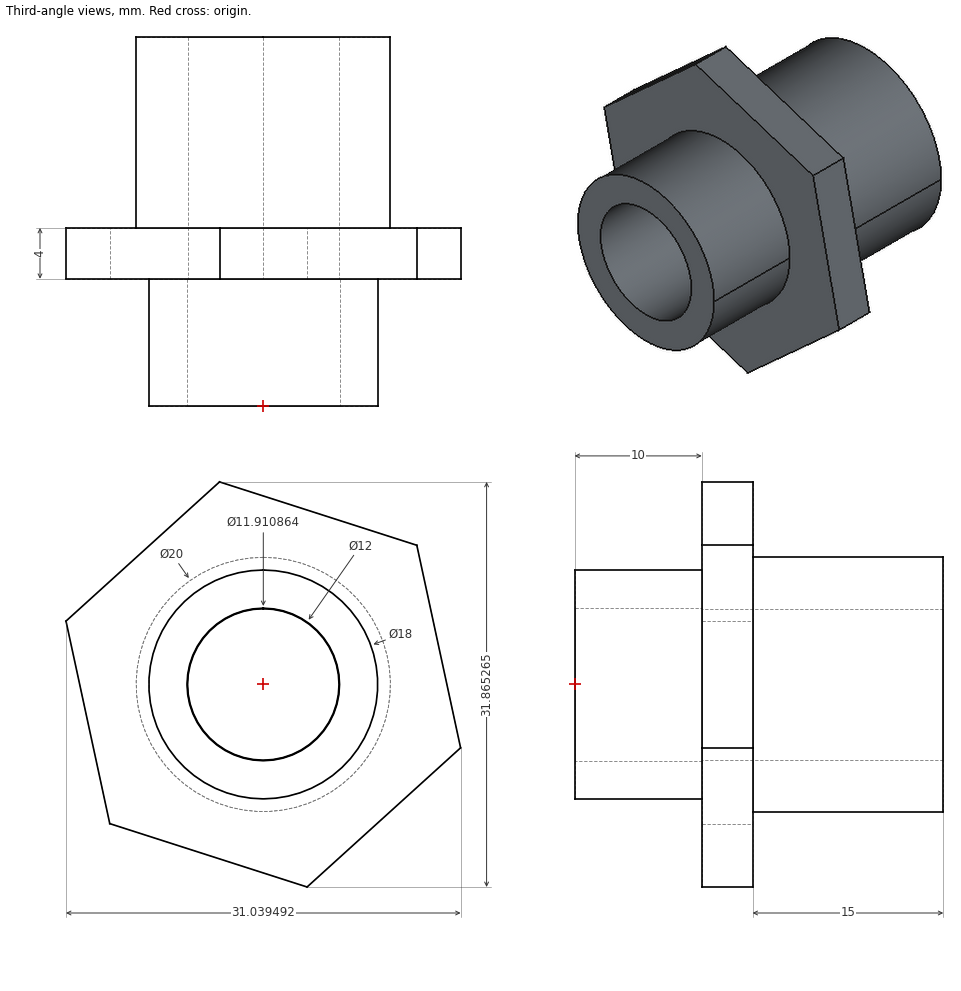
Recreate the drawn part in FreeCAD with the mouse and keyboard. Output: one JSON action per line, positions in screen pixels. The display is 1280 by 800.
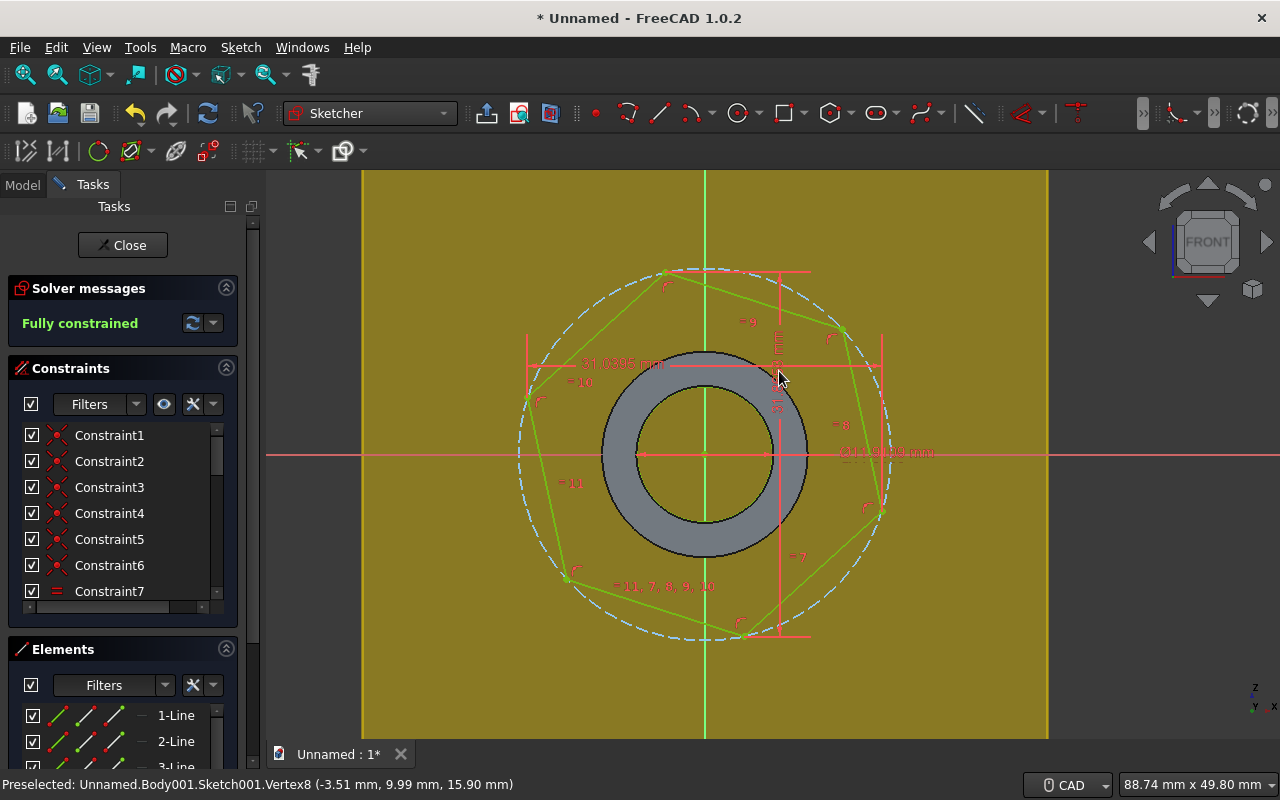
{"action": "left_click", "coordinate": [123, 245]}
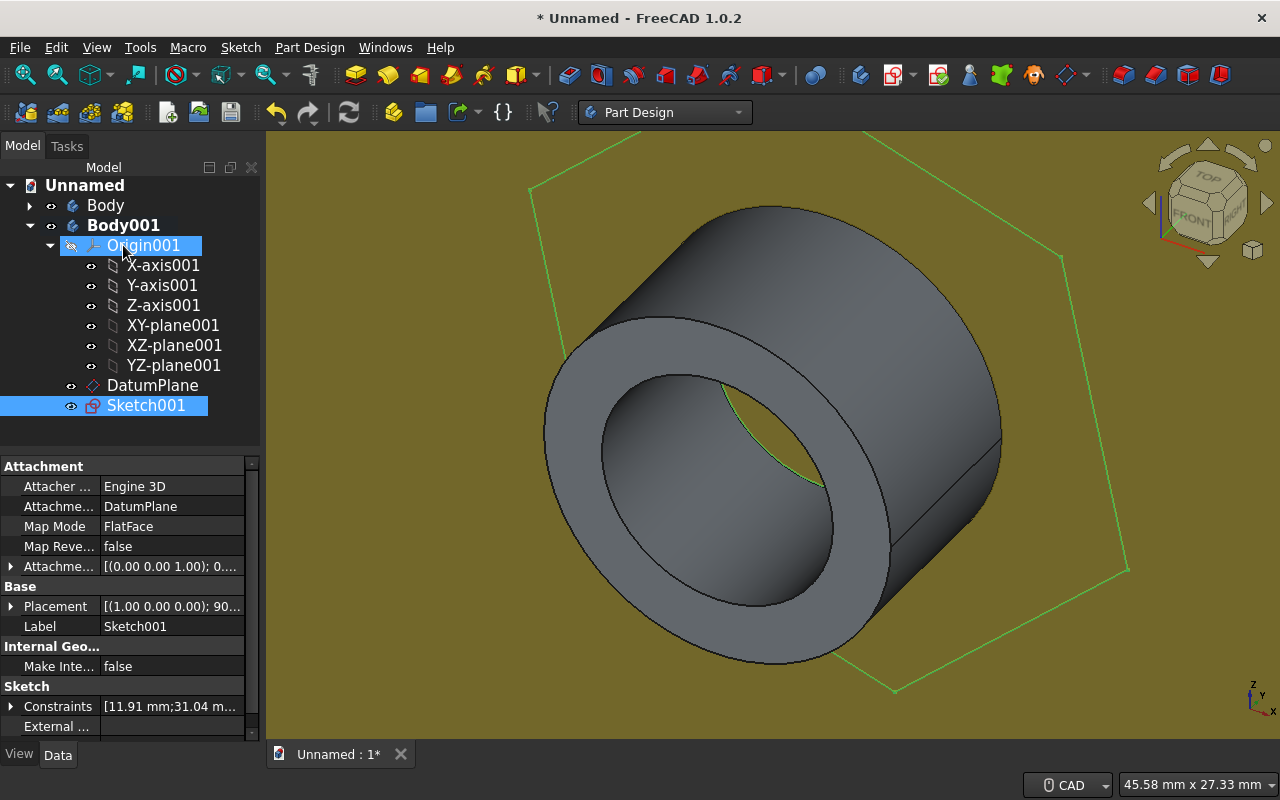
{"action": "left_click", "coordinate": [356, 76]}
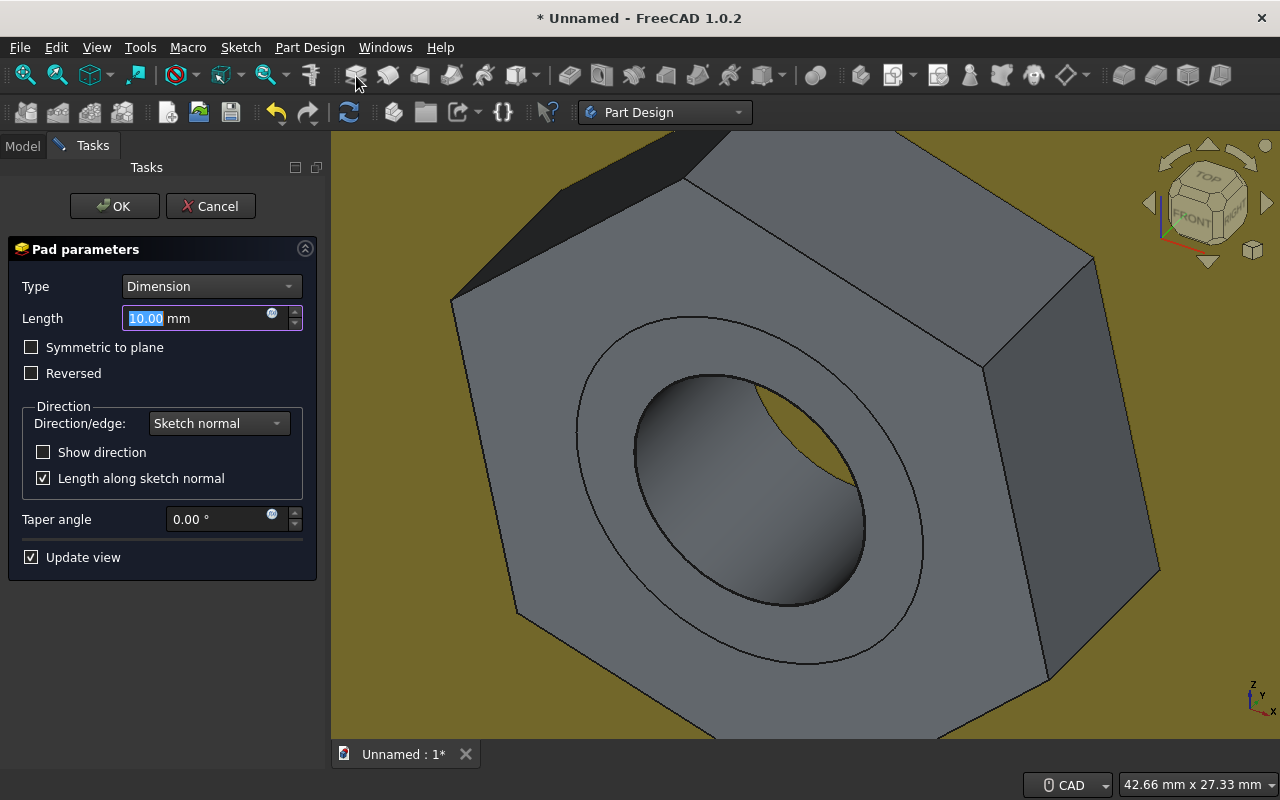
{"action": "type", "text": "4"}
{"action": "key", "text": "Tab"}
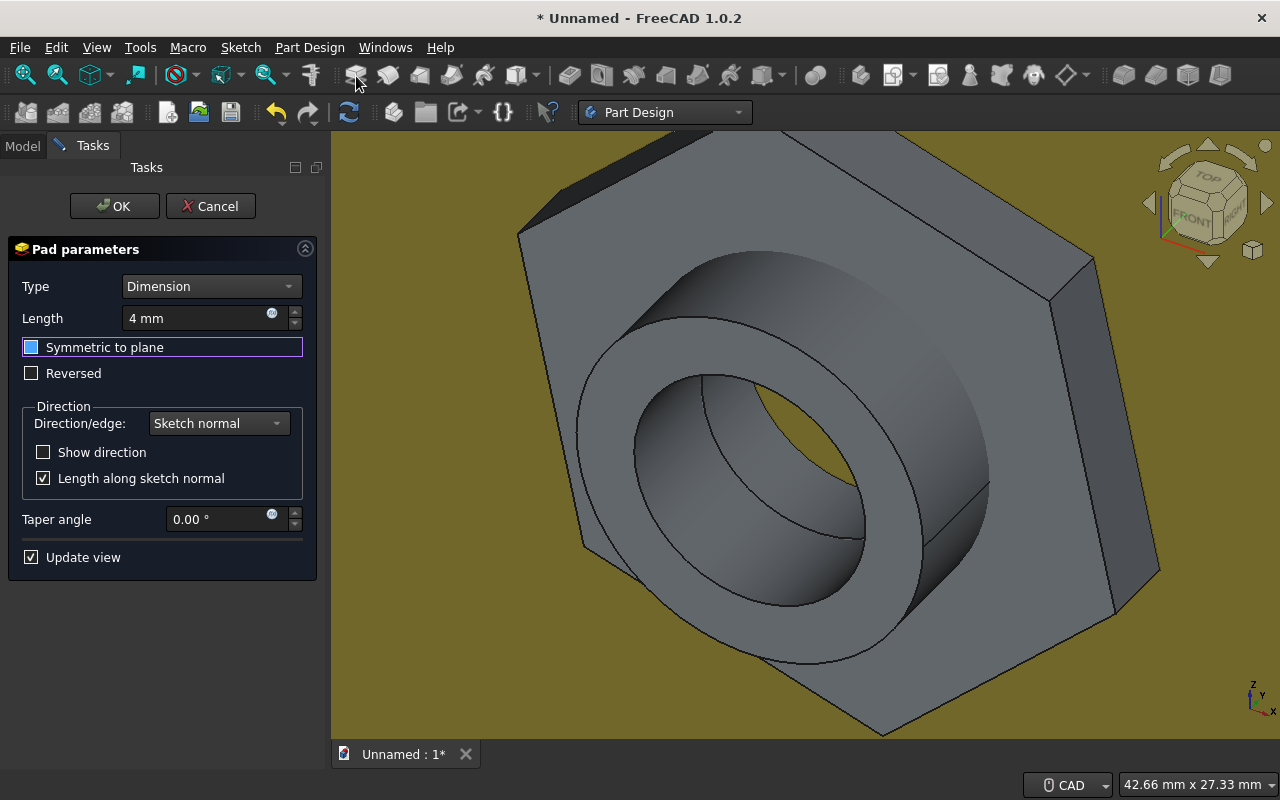
{"action": "left_click", "coordinate": [30, 373]}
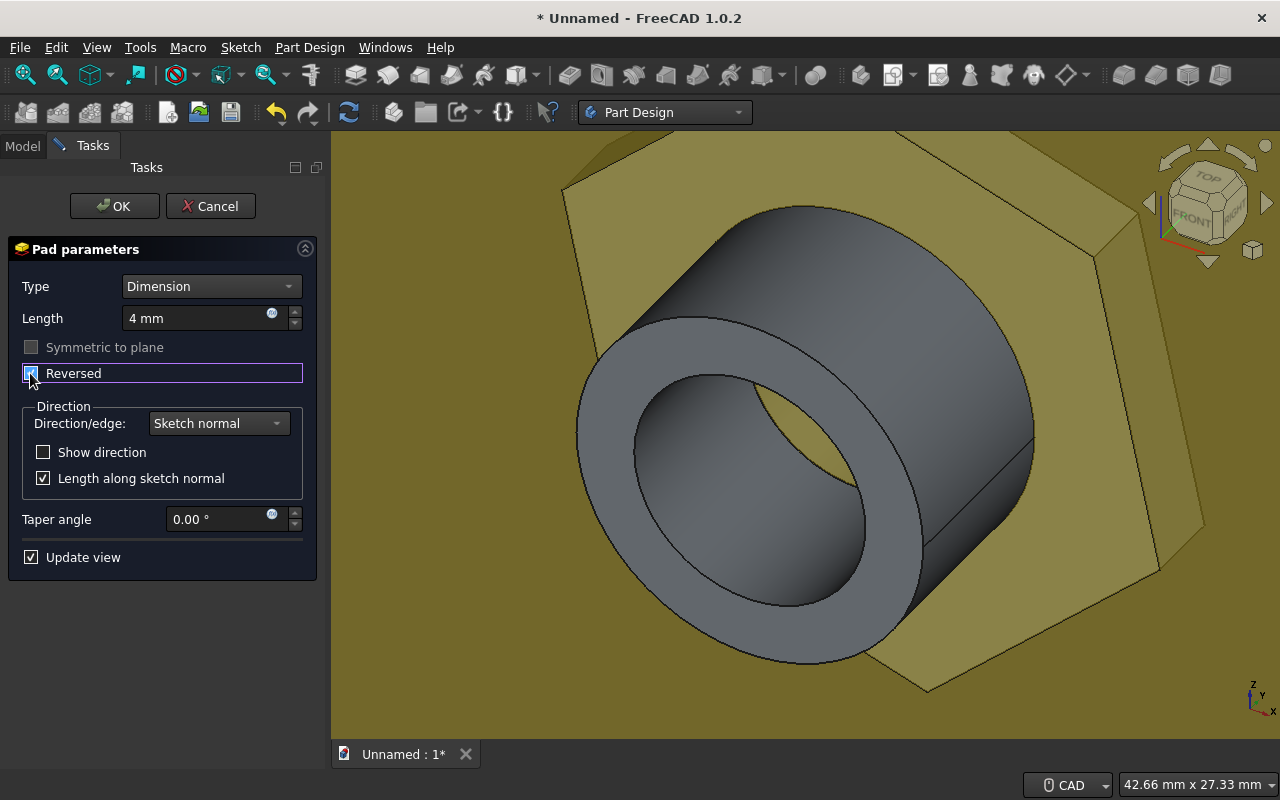
{"action": "left_click", "coordinate": [115, 206]}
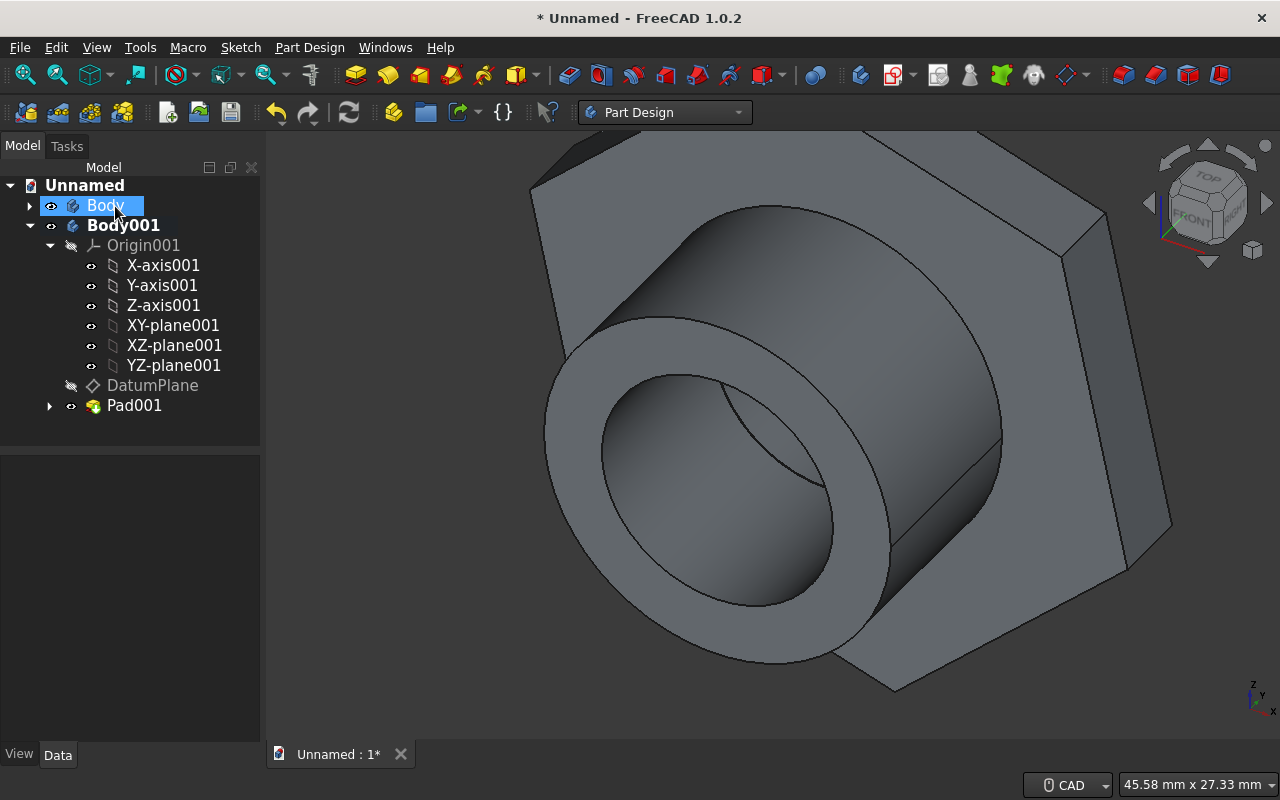
{"action": "left_click", "coordinate": [26, 76]}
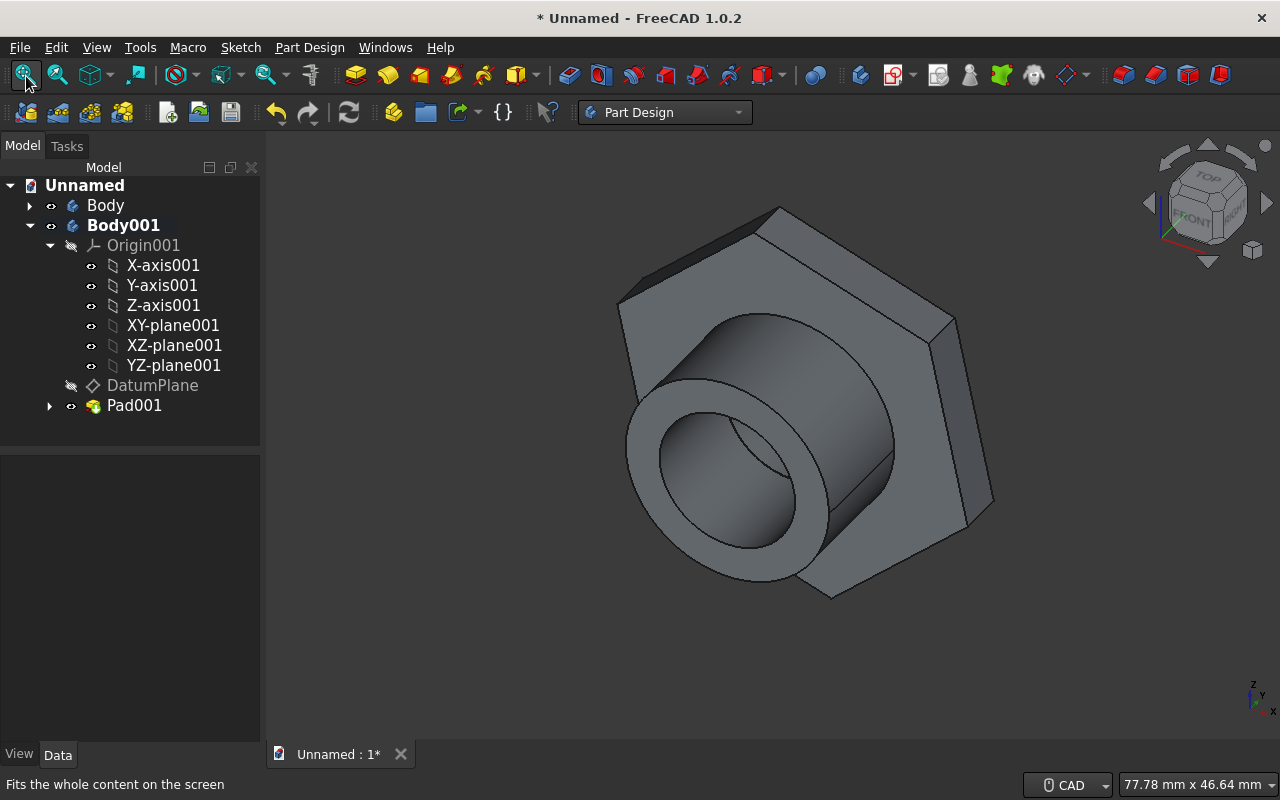
{"action": "key", "text": "4"}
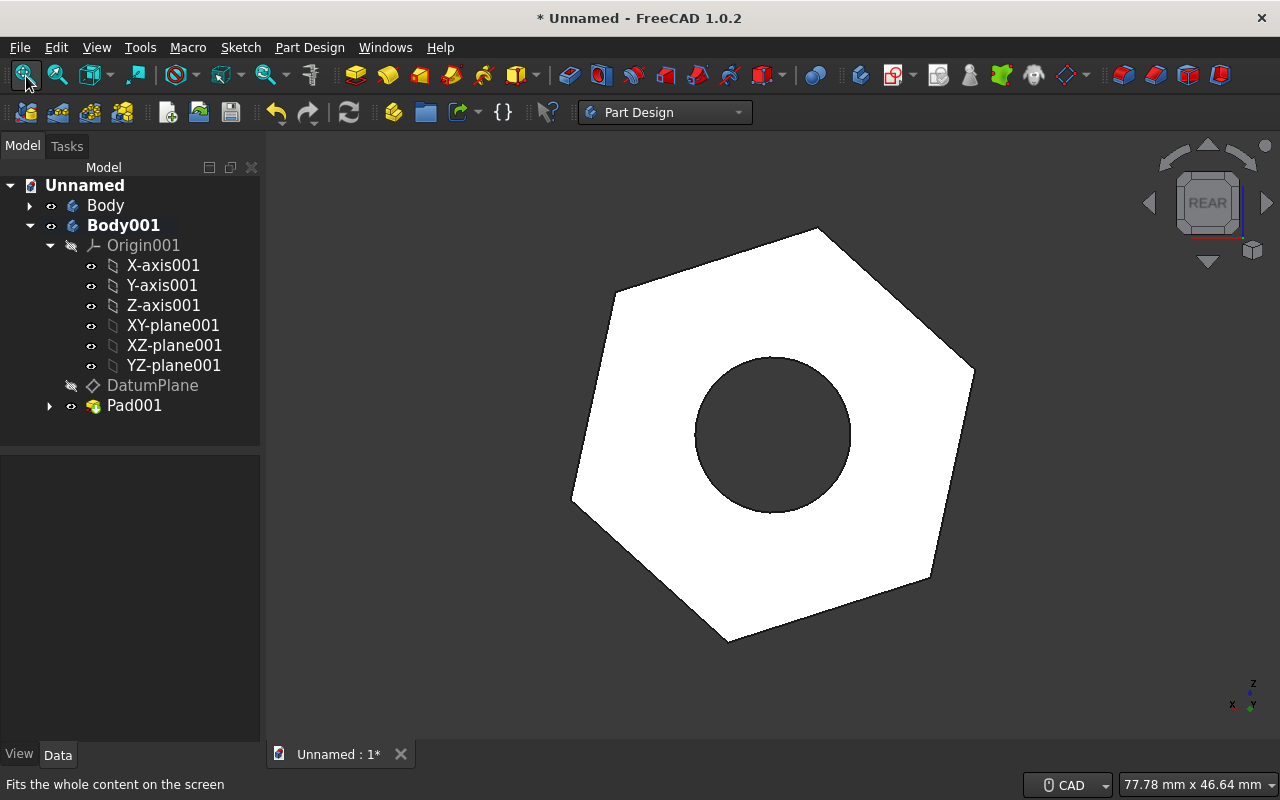
{"action": "left_click", "coordinate": [831, 315]}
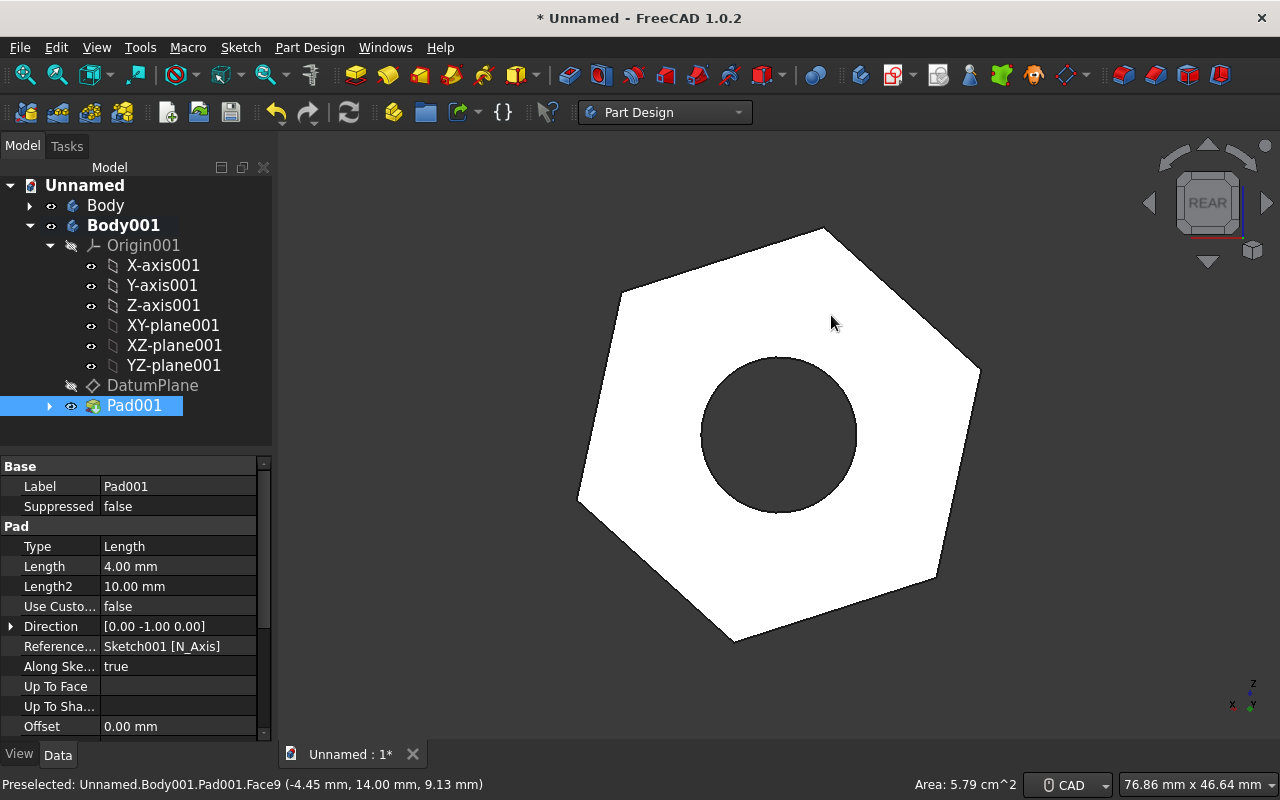
{"action": "left_click", "coordinate": [894, 76]}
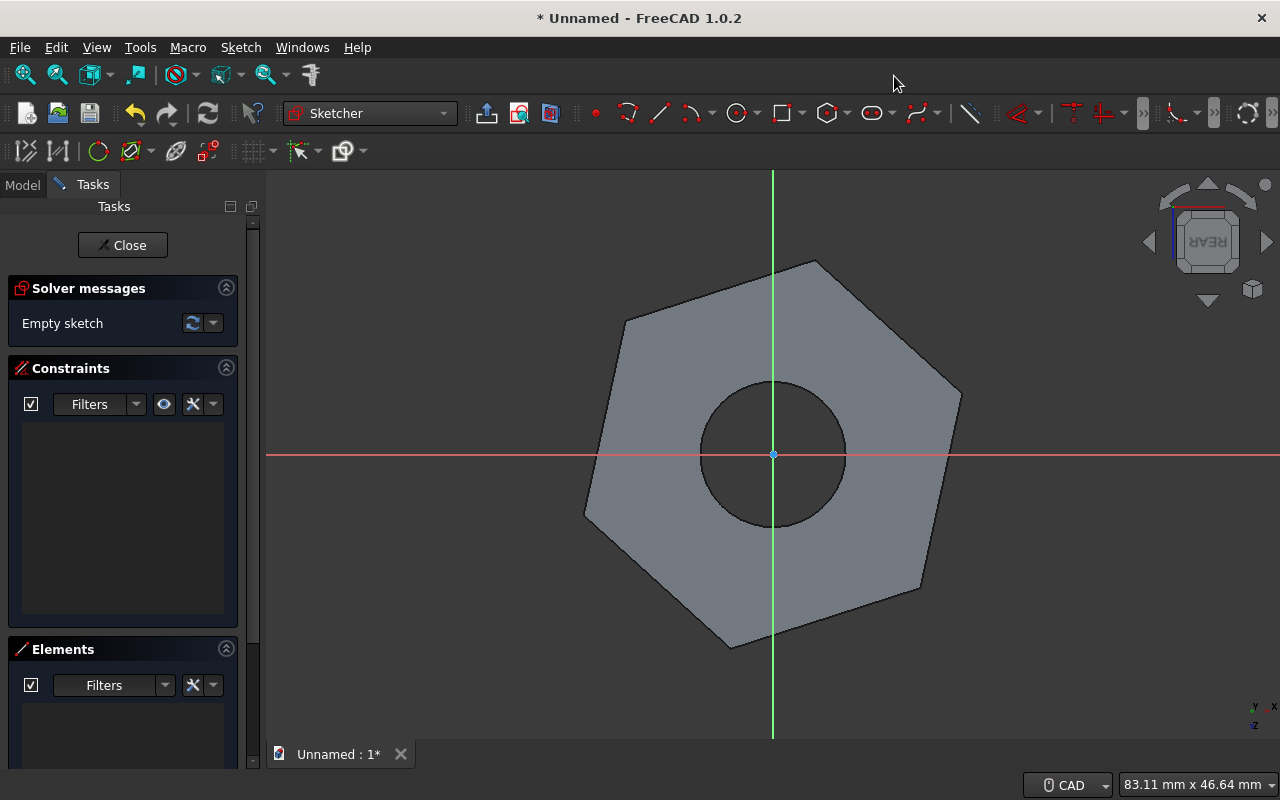
{"action": "scroll", "coordinate": [912, 455], "scroll_direction": "up", "scroll_amount": 2}